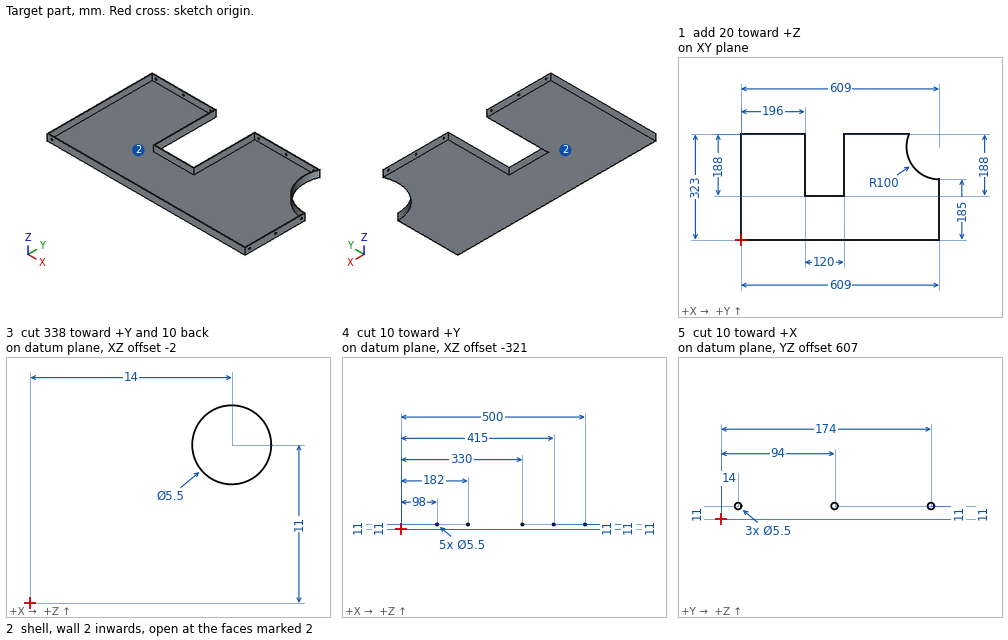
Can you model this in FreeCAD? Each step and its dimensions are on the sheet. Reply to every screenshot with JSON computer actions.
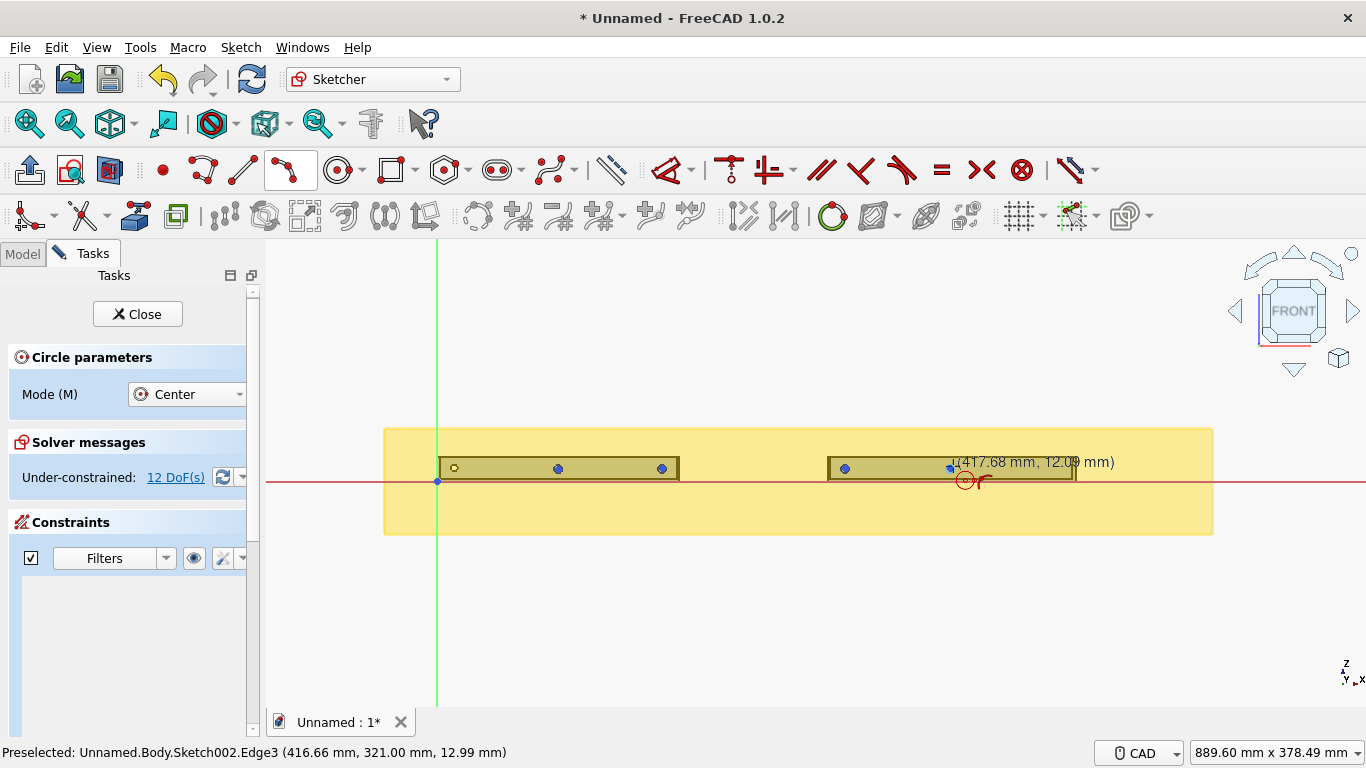
{"action": "scroll", "coordinate": [1055, 468], "scroll_direction": "up", "scroll_amount": 10}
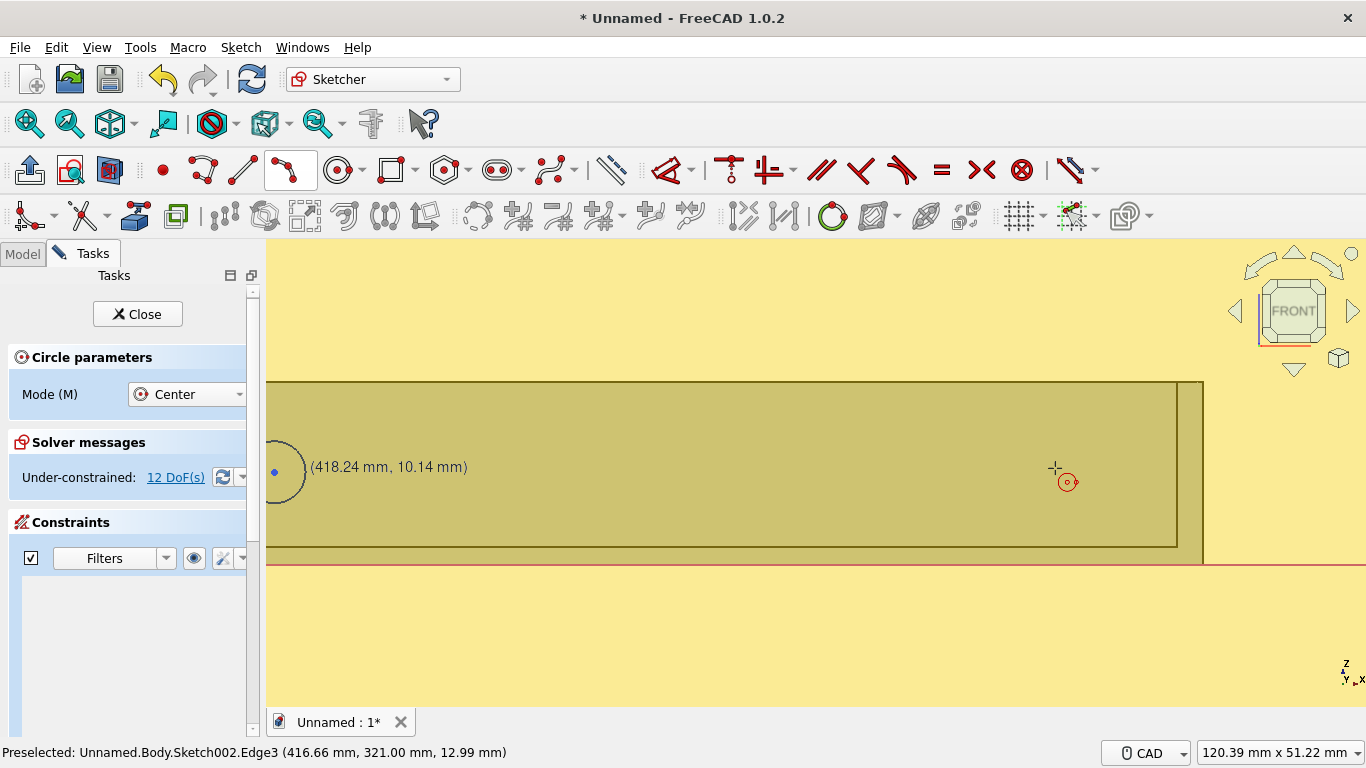
{"action": "scroll", "coordinate": [1055, 468], "scroll_direction": "down", "scroll_amount": 10}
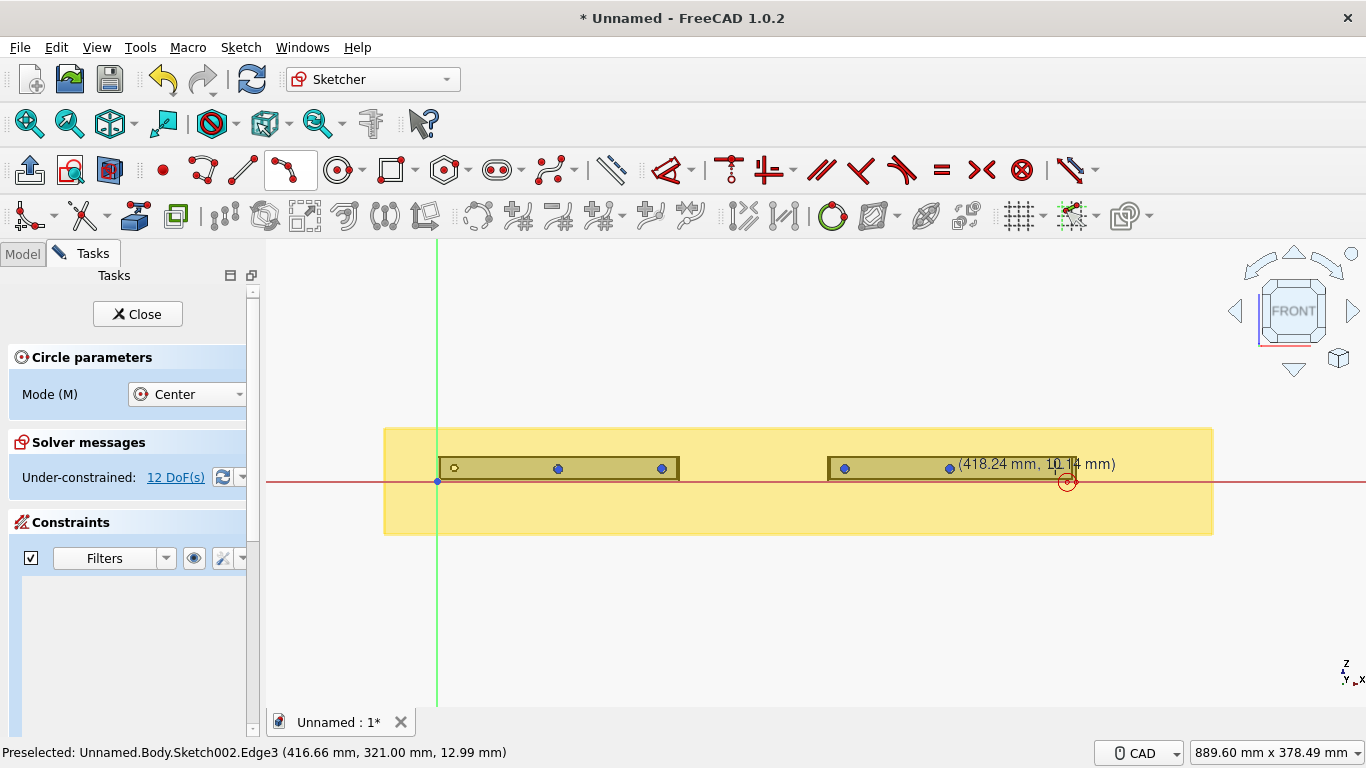
{"action": "left_click", "coordinate": [1055, 468]}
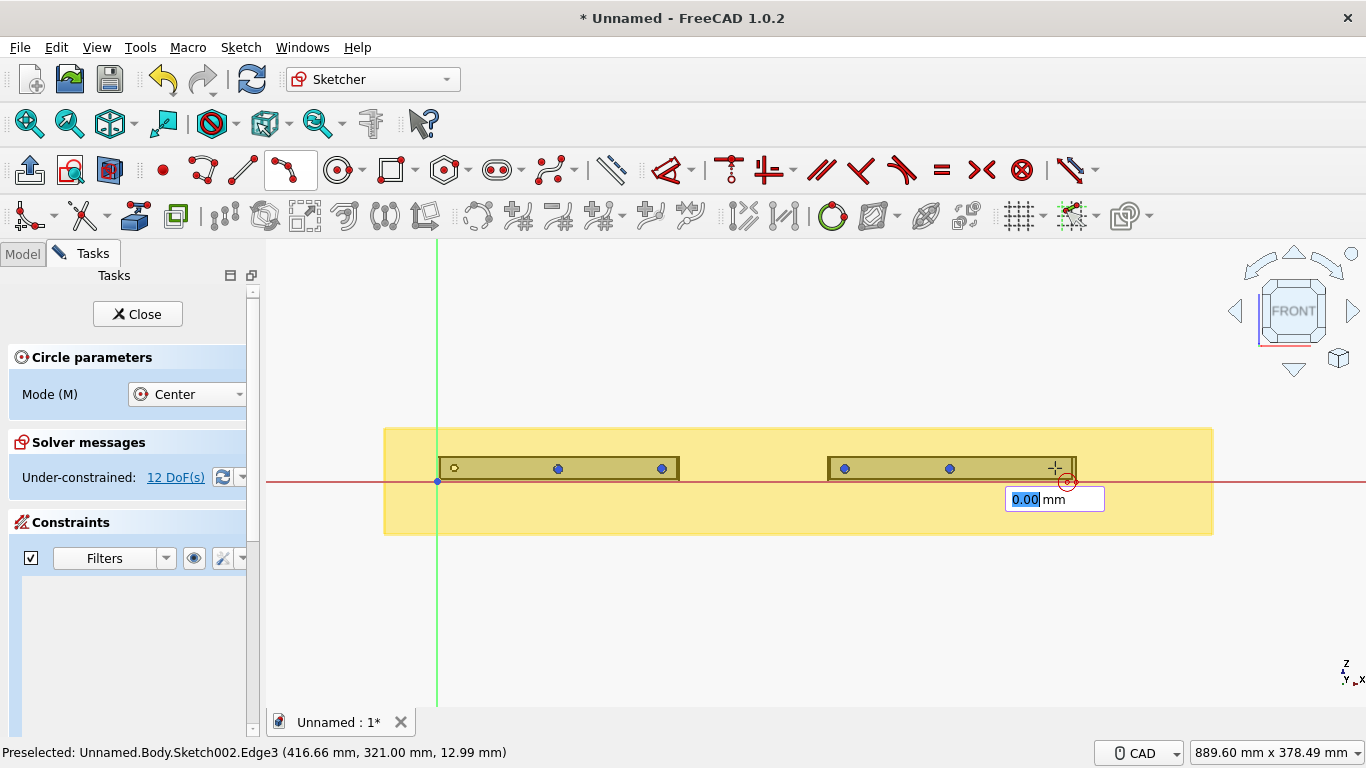
{"action": "scroll", "coordinate": [1058, 466], "scroll_direction": "up", "scroll_amount": 8}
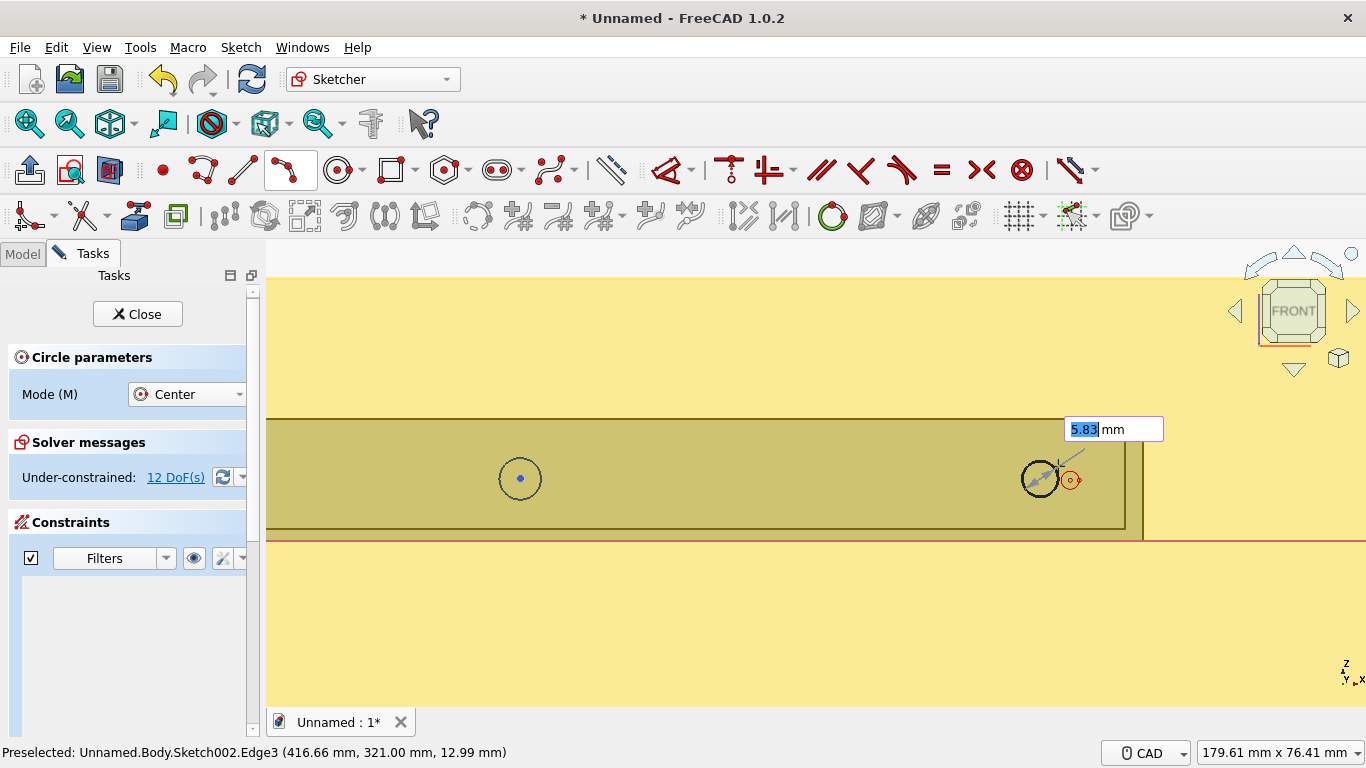
{"action": "left_click", "coordinate": [1054, 462]}
{"action": "key", "text": "Escape"}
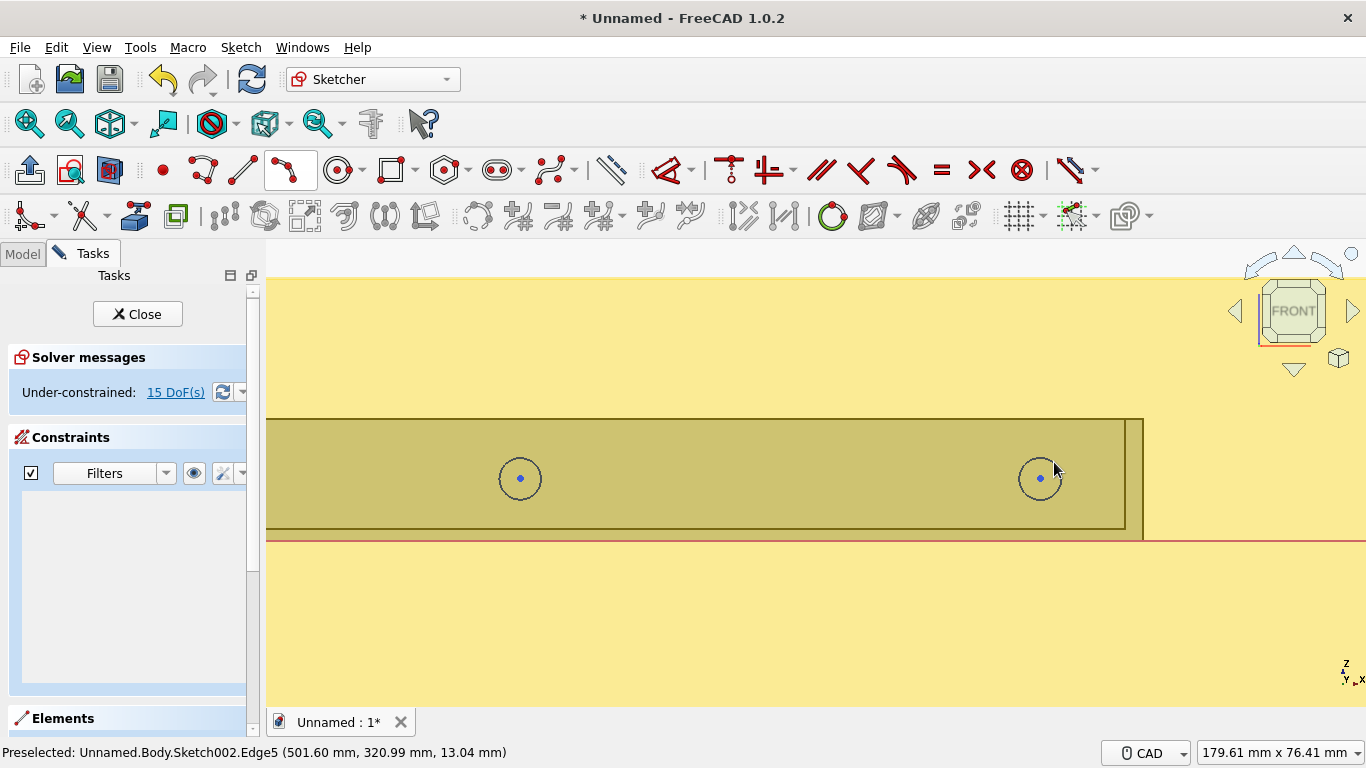
{"action": "scroll", "coordinate": [1058, 466], "scroll_direction": "down", "scroll_amount": 8}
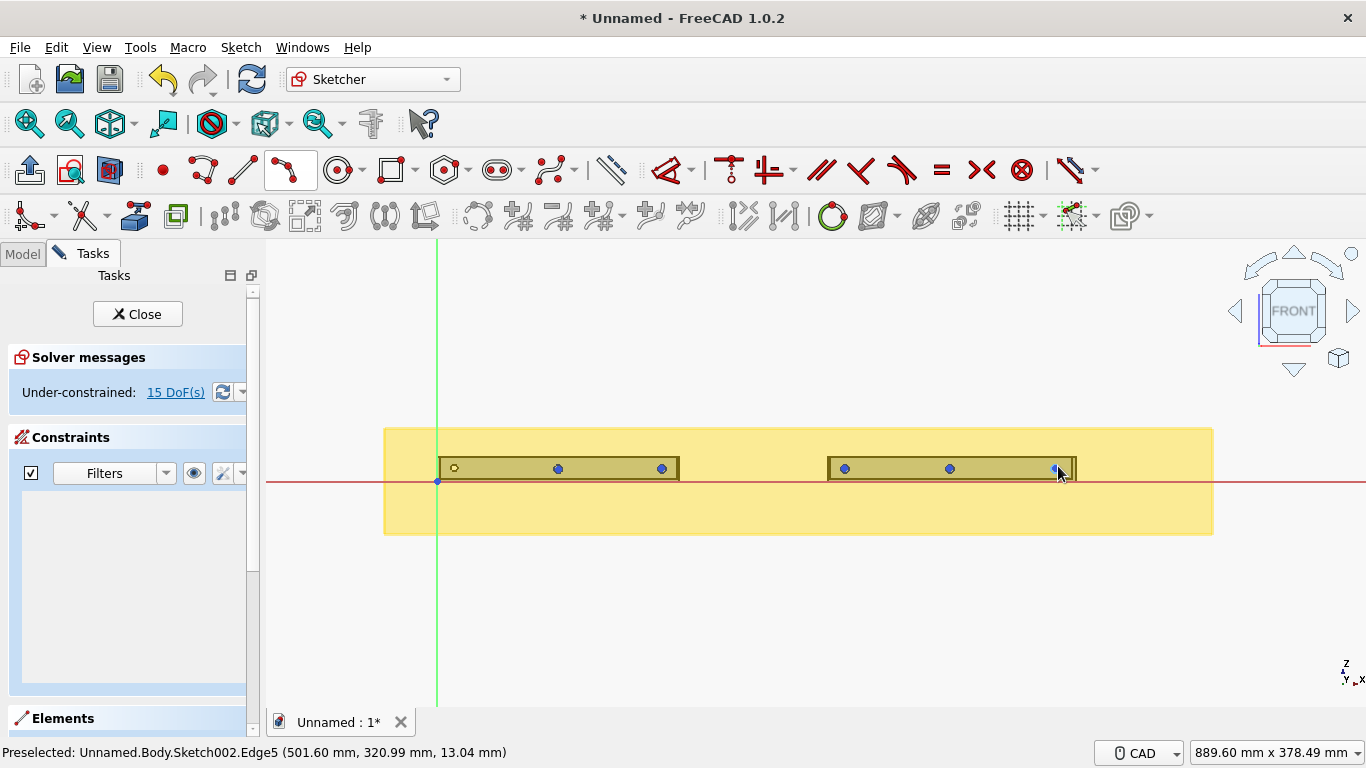
{"action": "scroll", "coordinate": [561, 466], "scroll_direction": "up", "scroll_amount": 6}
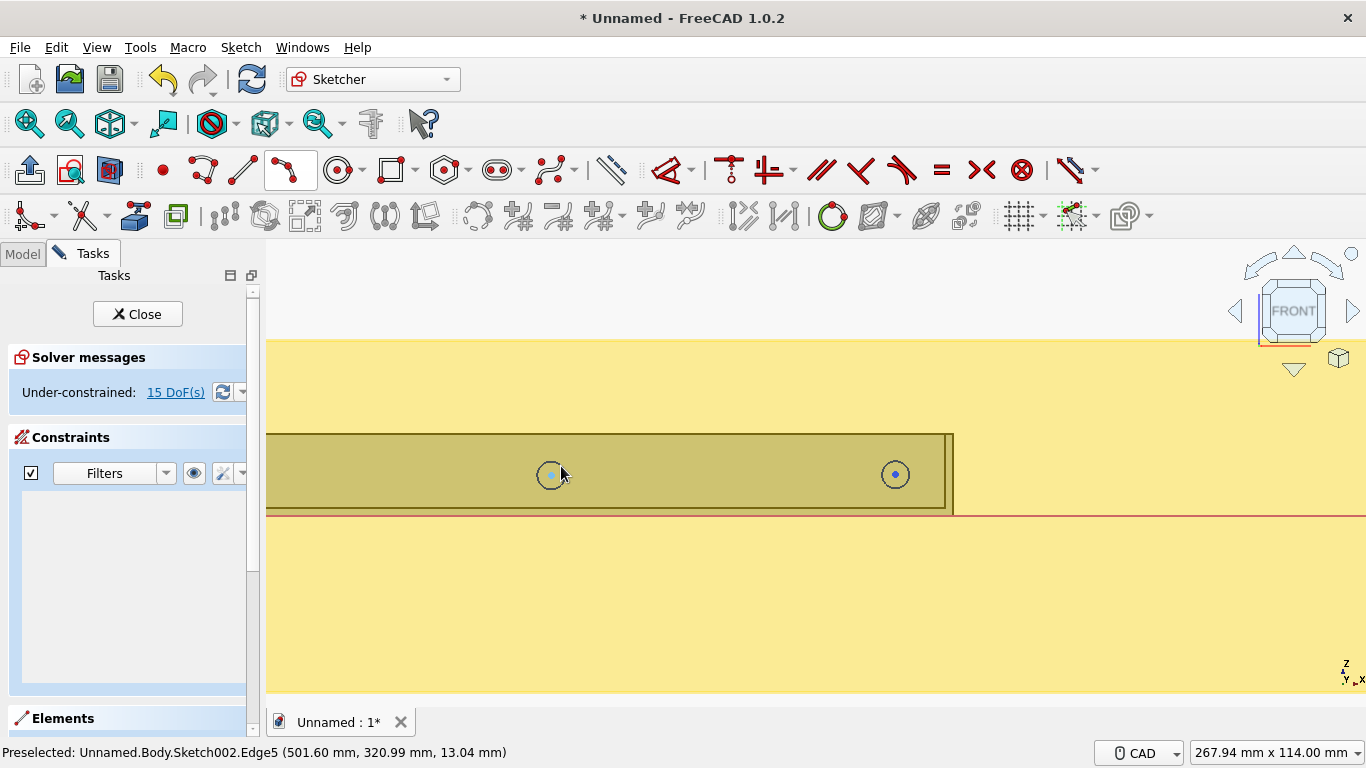
{"action": "left_click", "coordinate": [561, 466]}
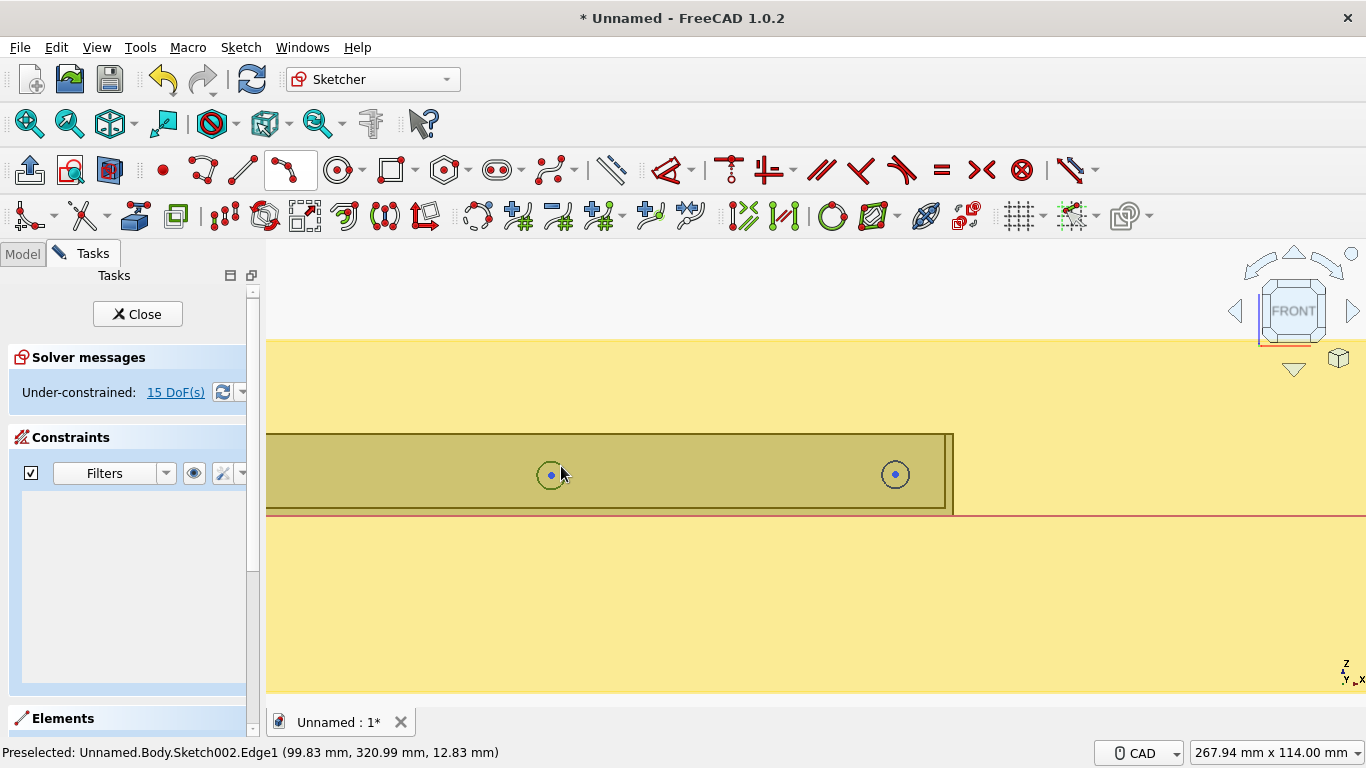
{"action": "left_click", "coordinate": [905, 465]}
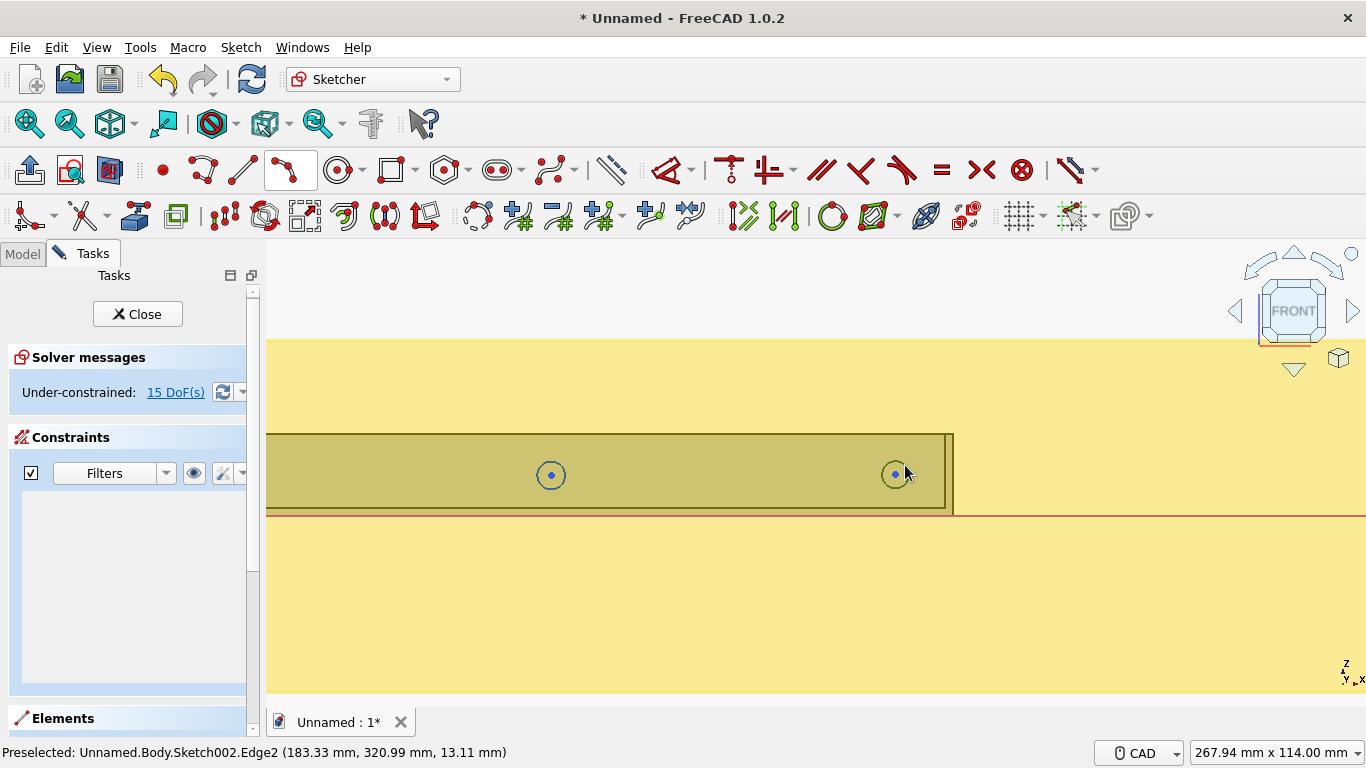
{"action": "scroll", "coordinate": [561, 466], "scroll_direction": "down", "scroll_amount": 6}